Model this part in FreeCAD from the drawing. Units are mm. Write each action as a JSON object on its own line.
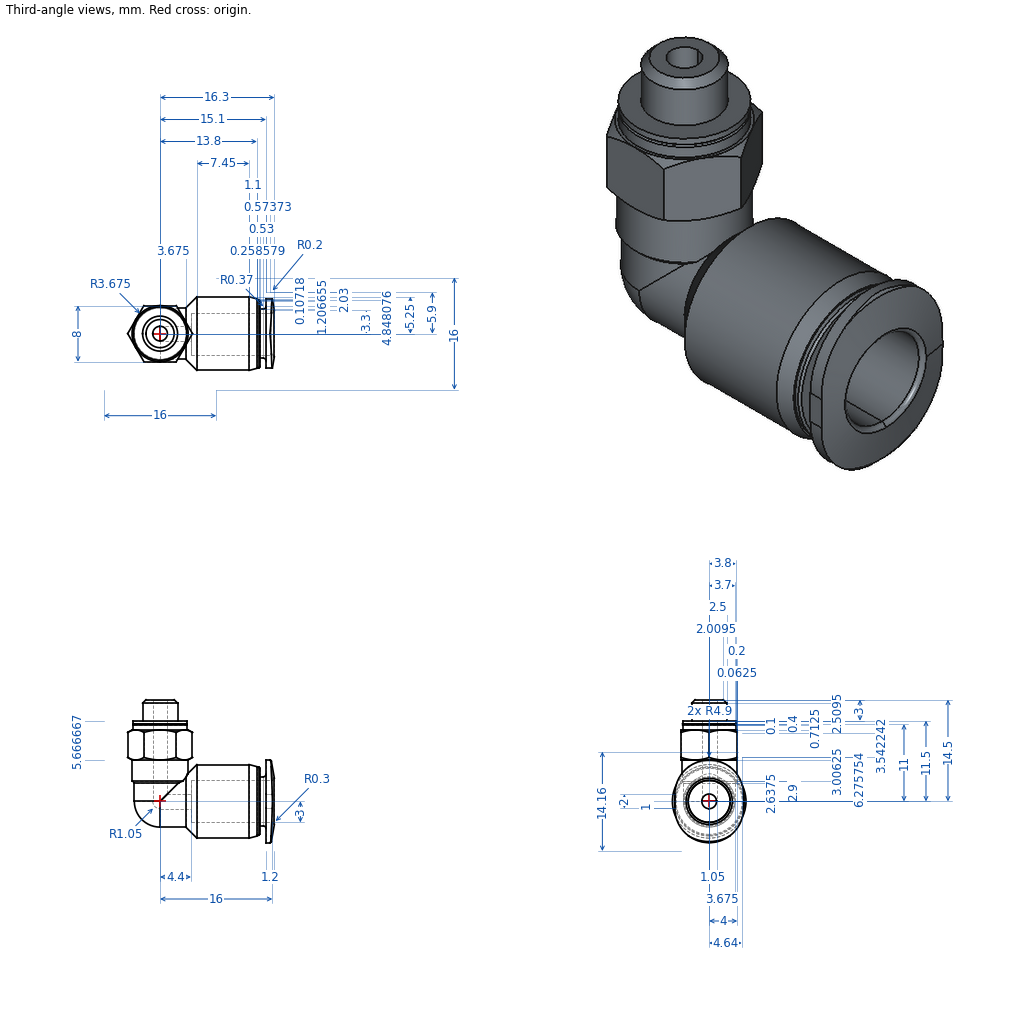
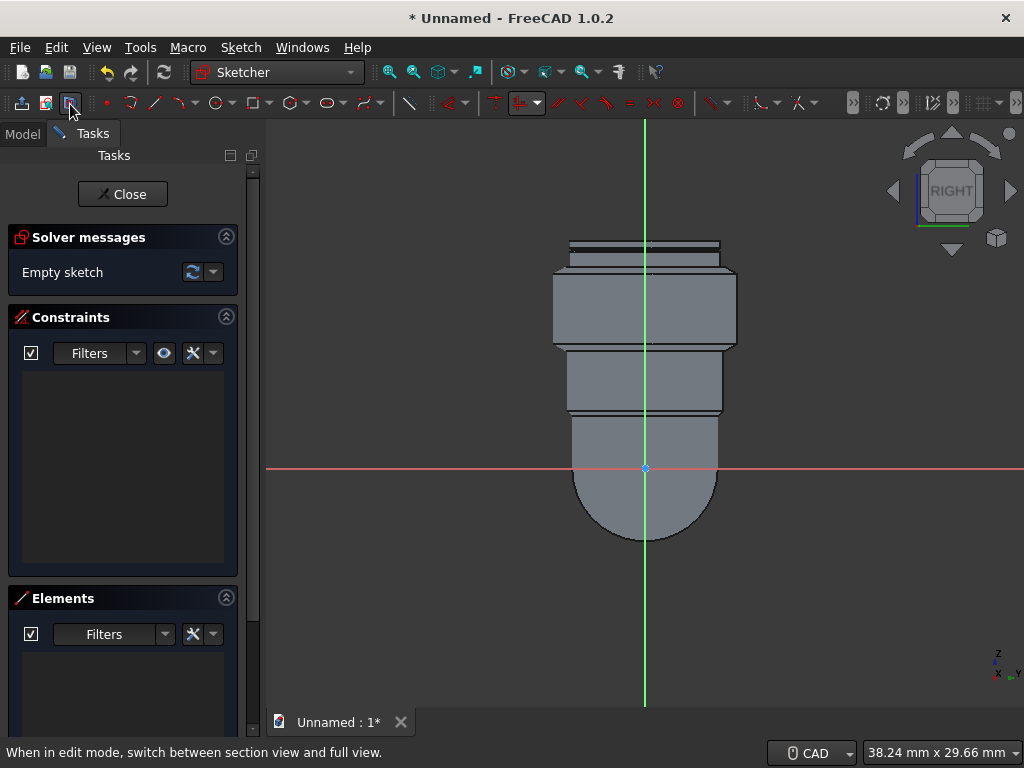
{"action": "scroll", "coordinate": [688, 171], "scroll_direction": "up", "scroll_amount": 9}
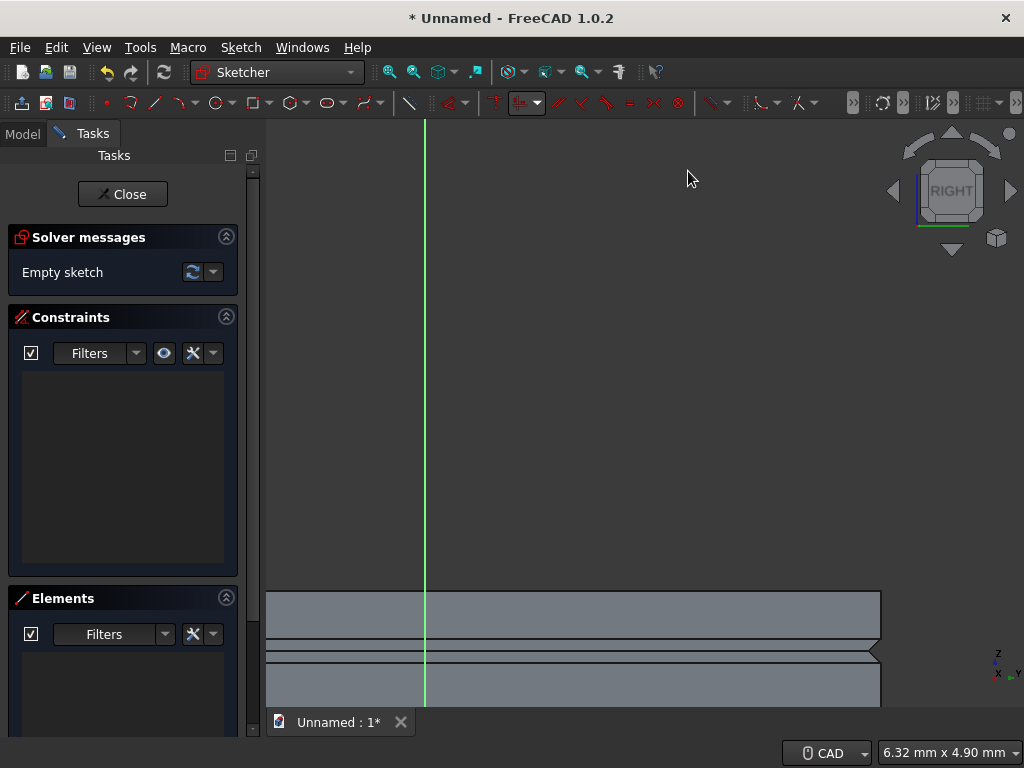
{"action": "left_click", "coordinate": [132, 104]}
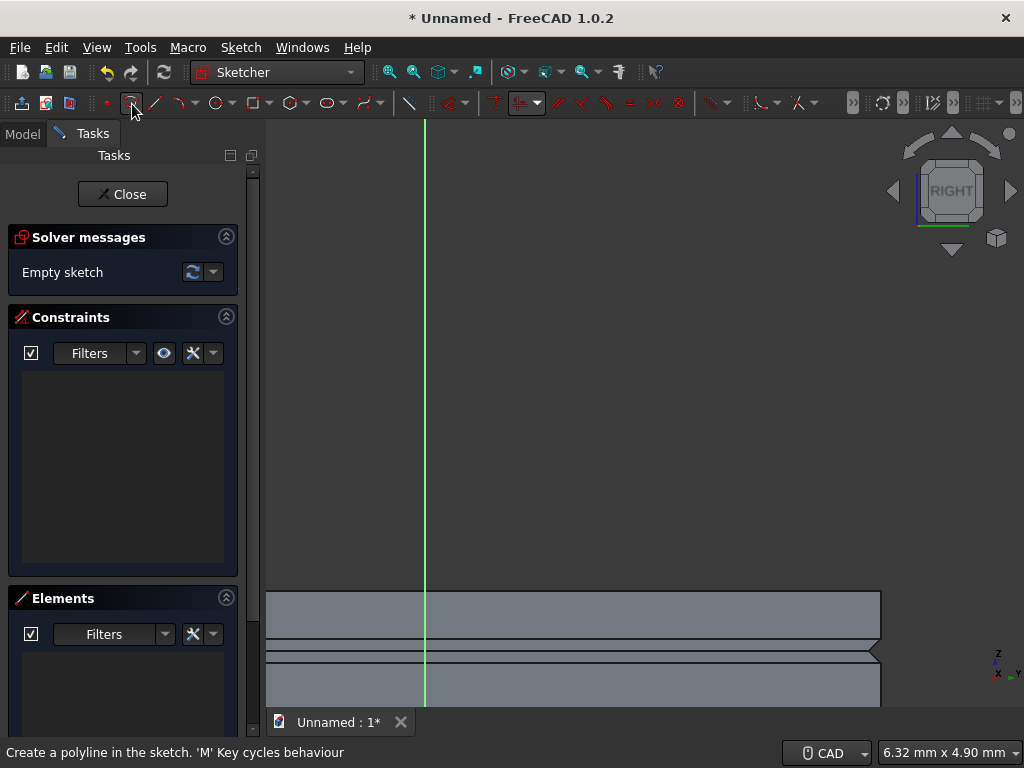
{"action": "left_click", "coordinate": [425, 591]}
{"action": "left_click", "coordinate": [725, 591]}
{"action": "left_click", "coordinate": [725, 290]}
{"action": "left_click", "coordinate": [666, 231]}
{"action": "left_click", "coordinate": [434, 231]}
{"action": "left_click", "coordinate": [425, 592]}
{"action": "key", "text": "Escape"}
{"action": "key", "text": "Escape"}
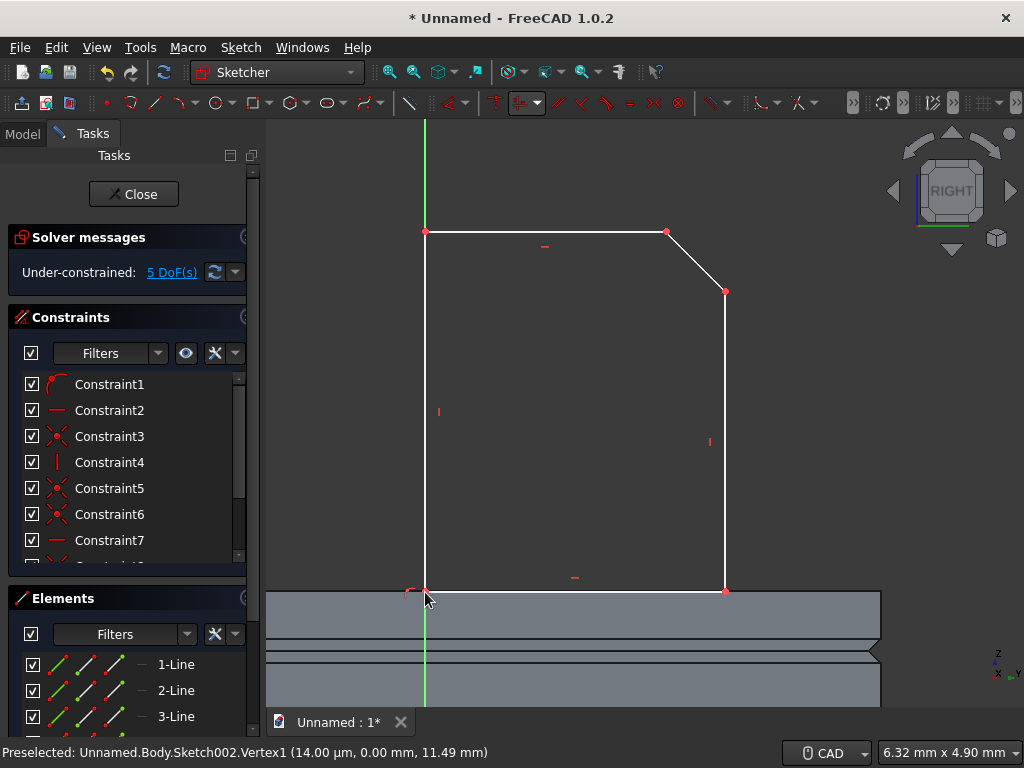
{"action": "left_click", "coordinate": [448, 104]}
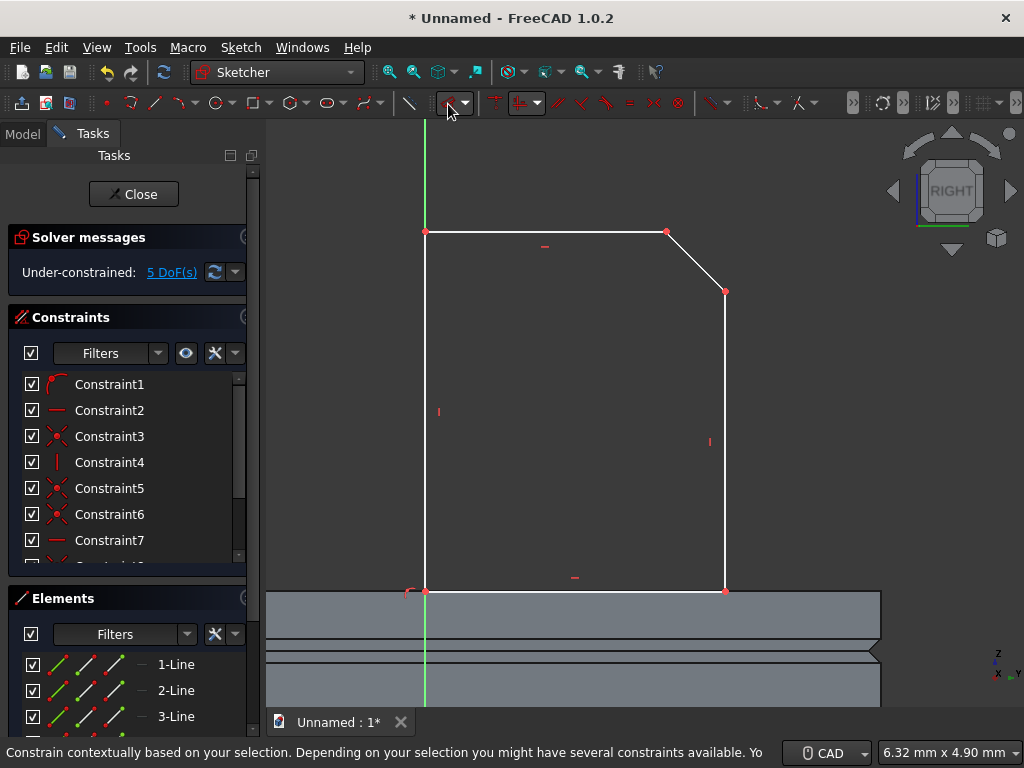
{"action": "left_click", "coordinate": [425, 340]}
{"action": "left_click", "coordinate": [391, 412]}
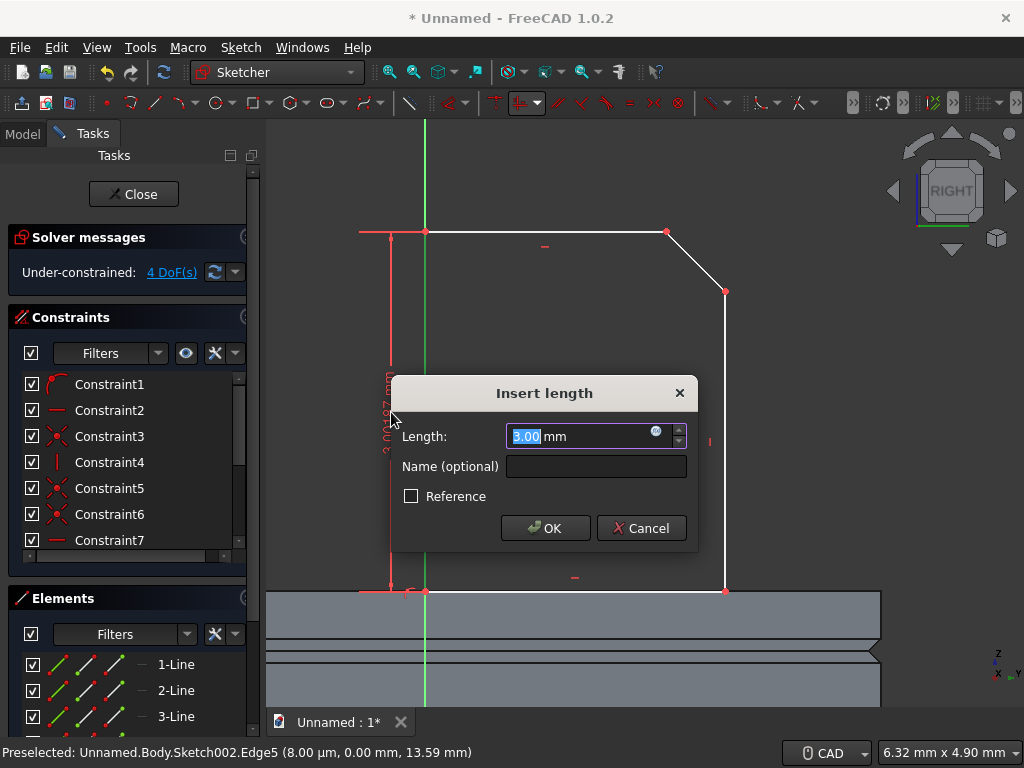
{"action": "type", "text": "3"}
{"action": "key", "text": "Return"}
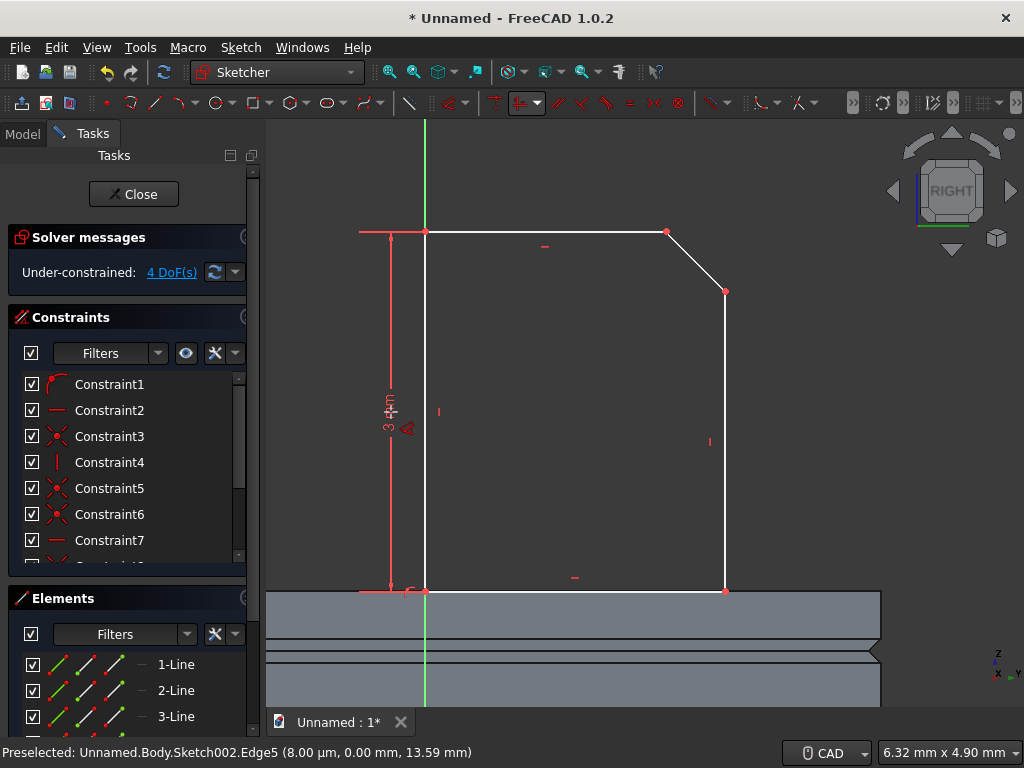
{"action": "left_click", "coordinate": [515, 592]}
{"action": "left_click", "coordinate": [575, 626]}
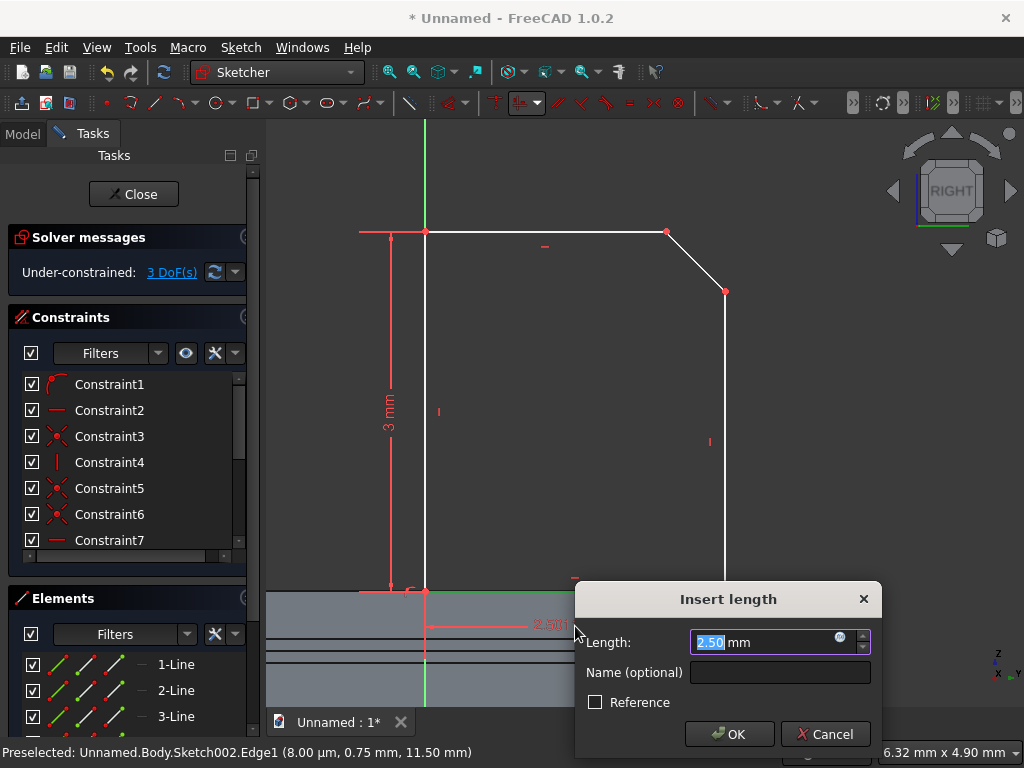
{"action": "type", "text": "2.5"}
{"action": "key", "text": "Return"}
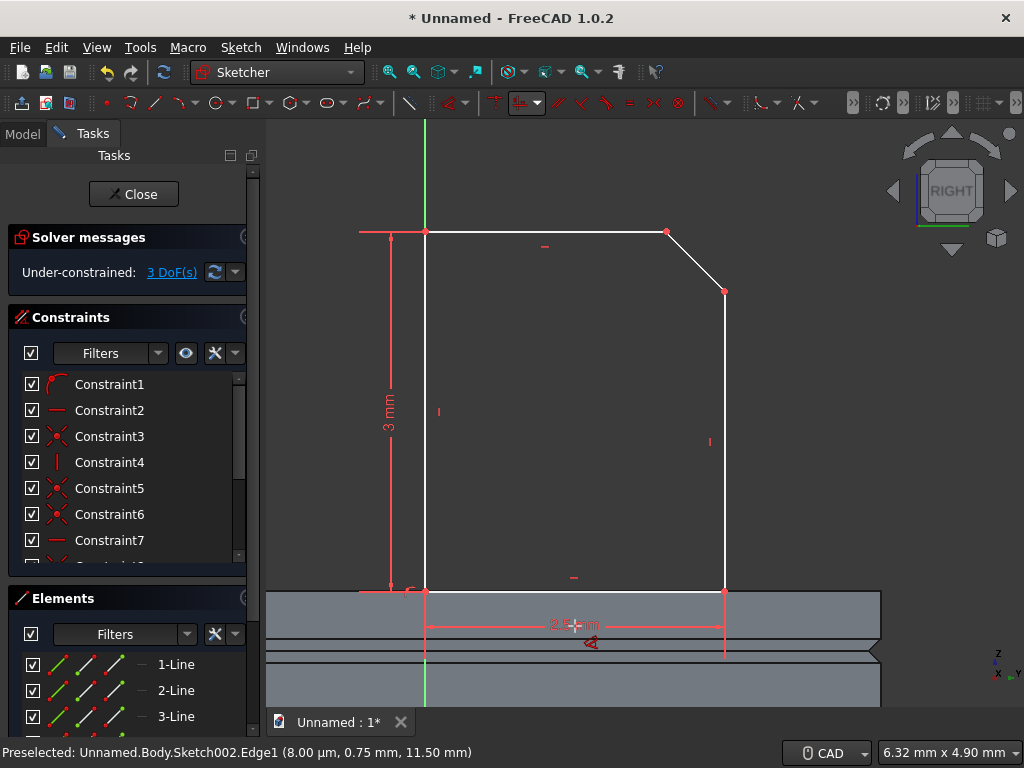
{"action": "left_click", "coordinate": [425, 592]}
{"action": "left_click", "coordinate": [391, 635]}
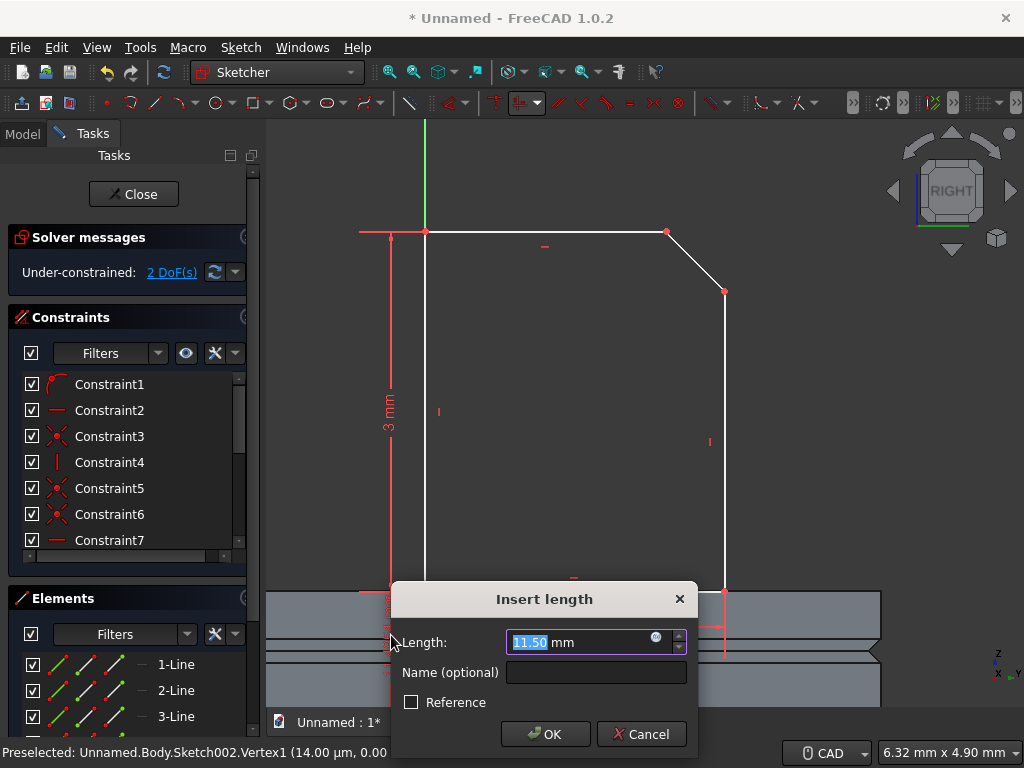
{"action": "type", "text": "11.5"}
{"action": "key", "text": "Return"}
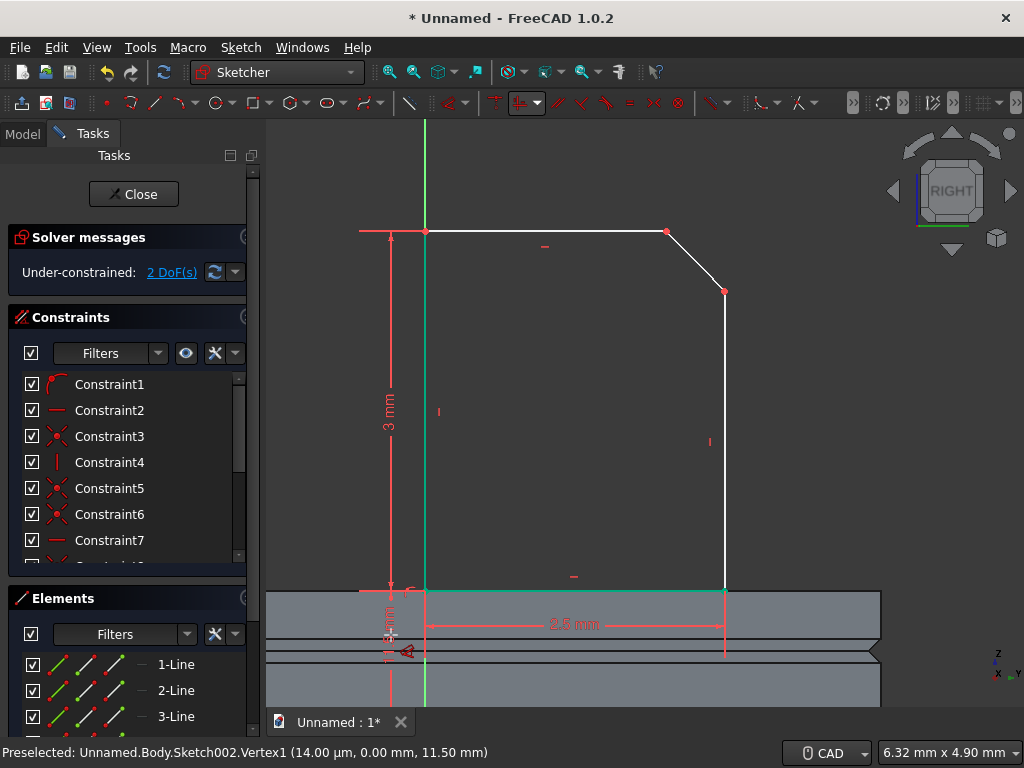
{"action": "left_click", "coordinate": [725, 501]}
{"action": "left_click", "coordinate": [759, 441]}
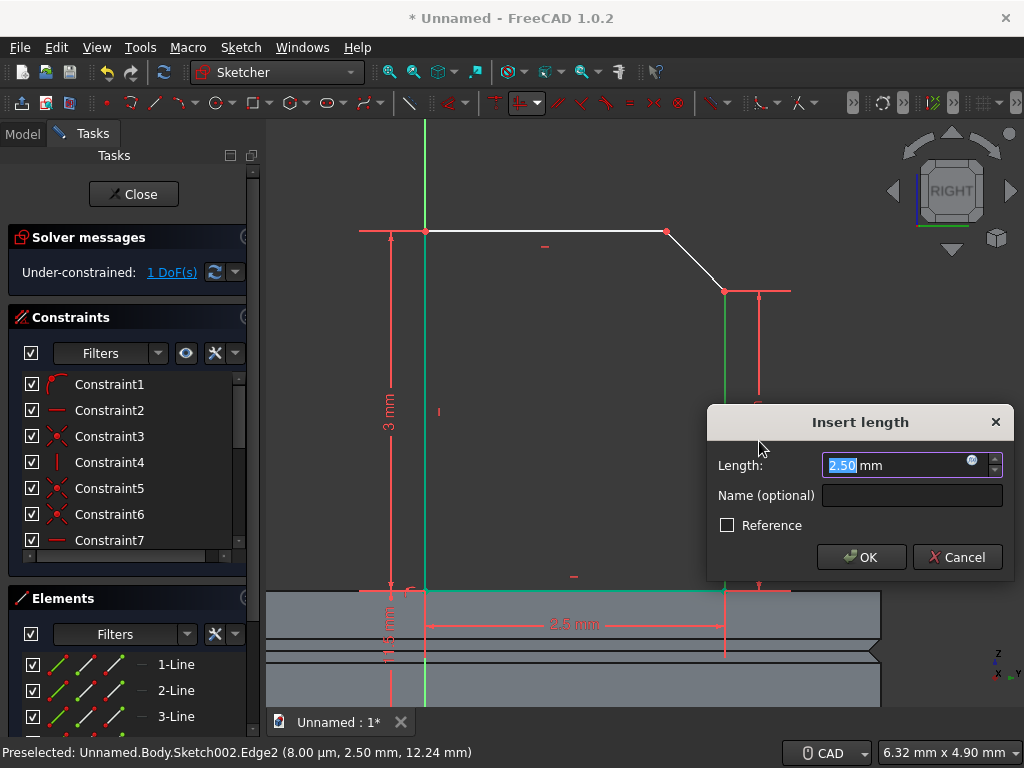
{"action": "type", "text": "2.5095"}
{"action": "key", "text": "Return"}